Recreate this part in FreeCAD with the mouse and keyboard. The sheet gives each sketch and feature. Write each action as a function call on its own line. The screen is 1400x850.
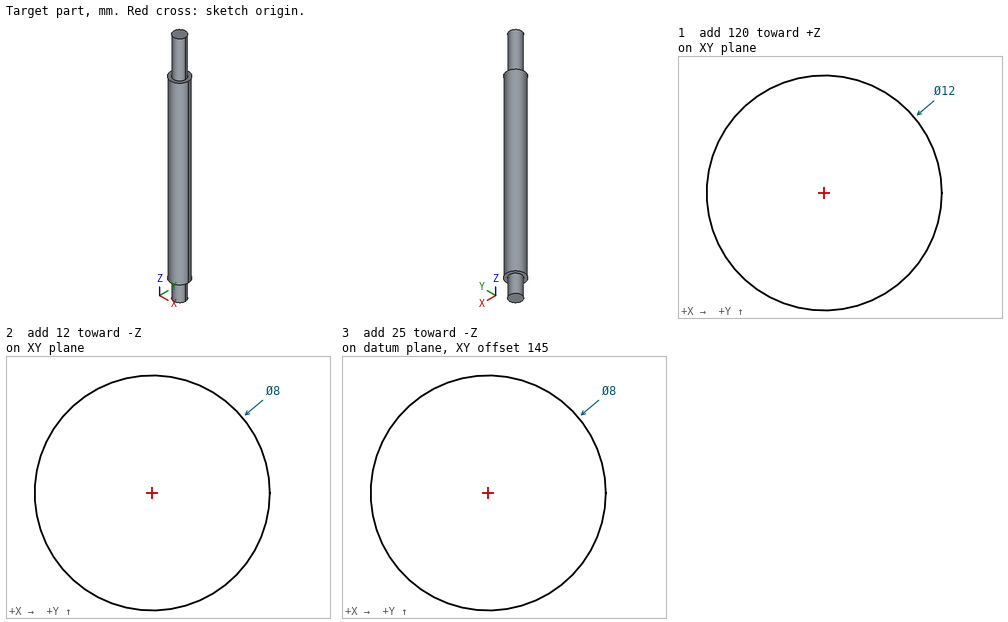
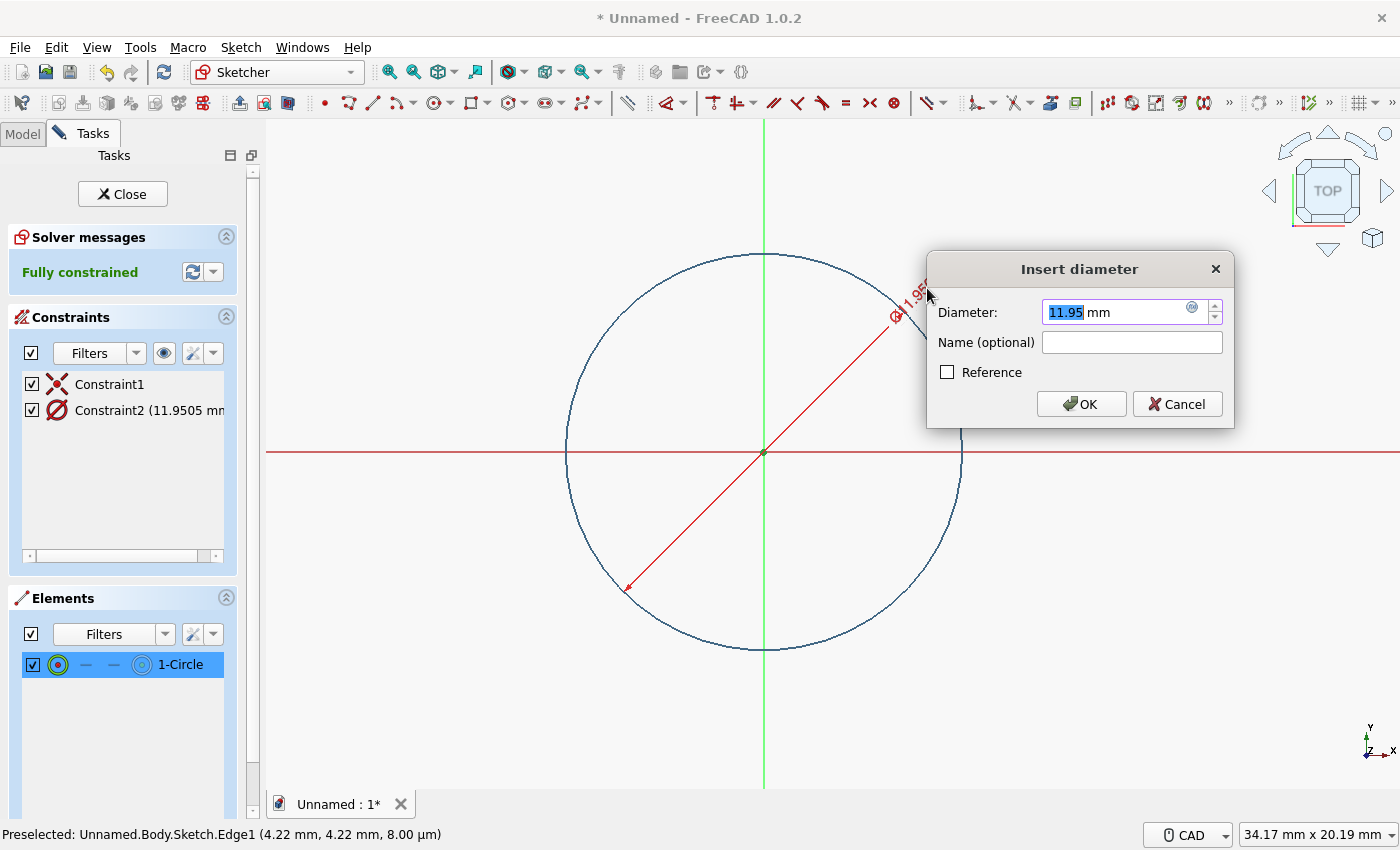
text(12)
key(Return)
key(Escape)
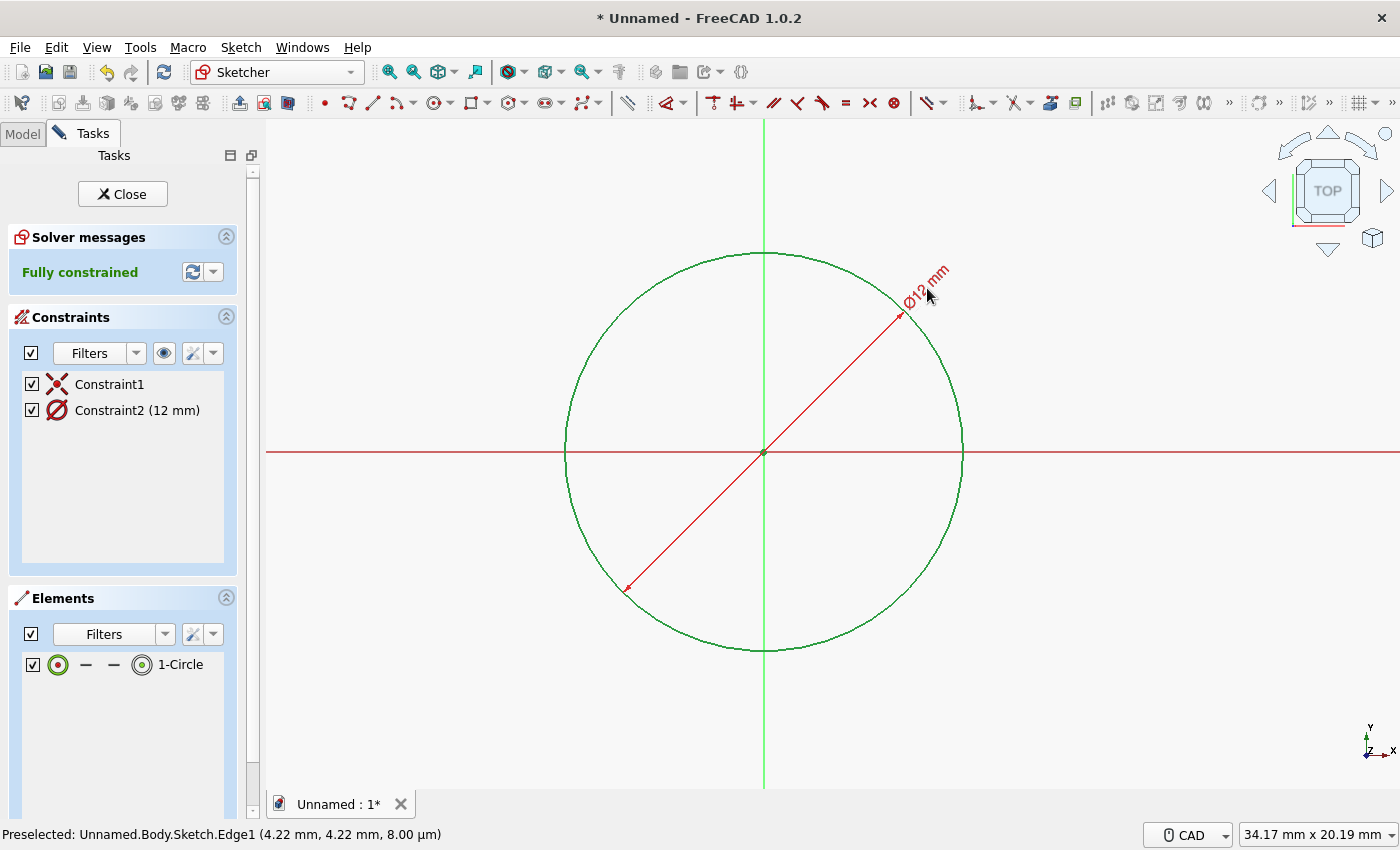
click(123, 194)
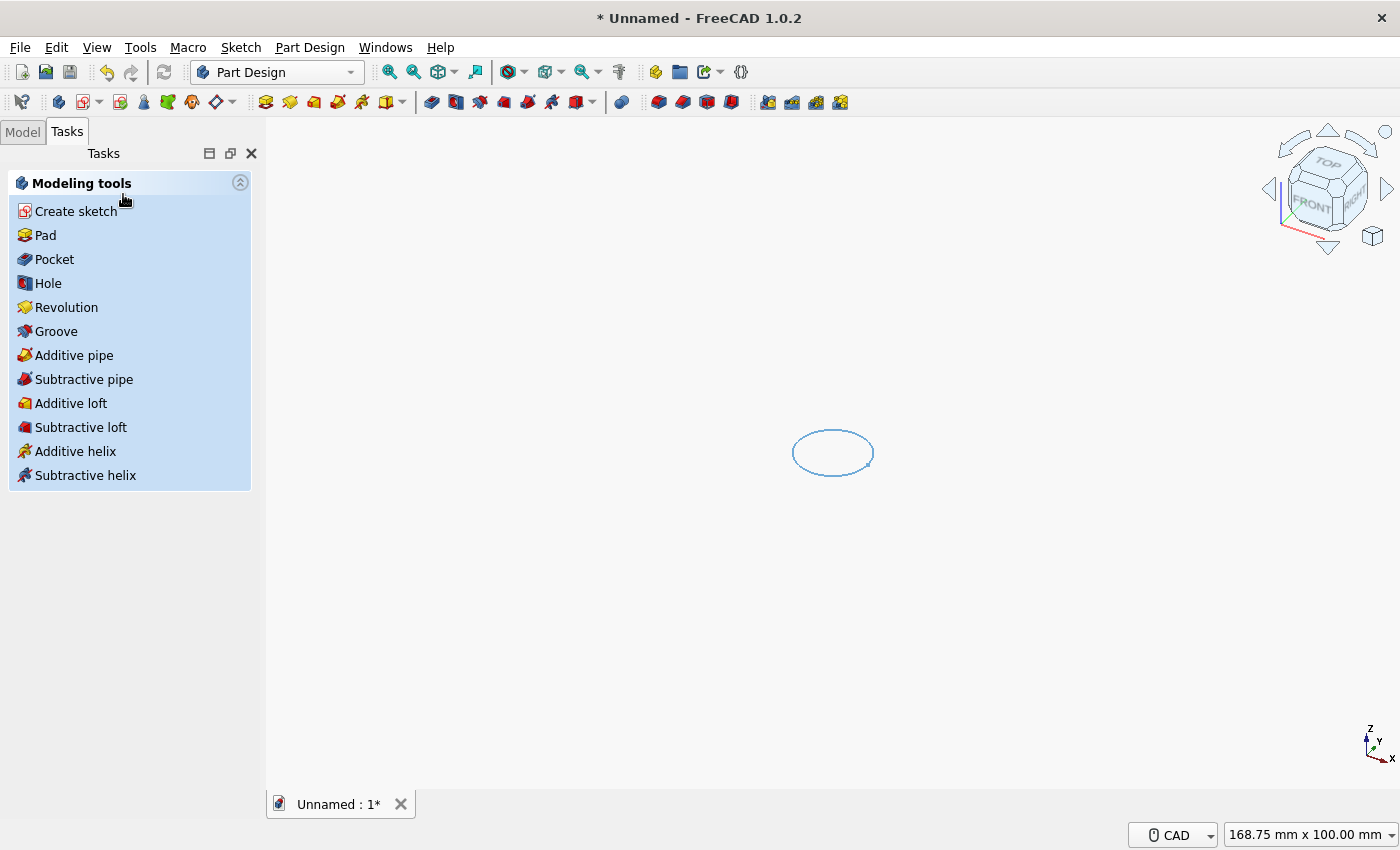
click(266, 102)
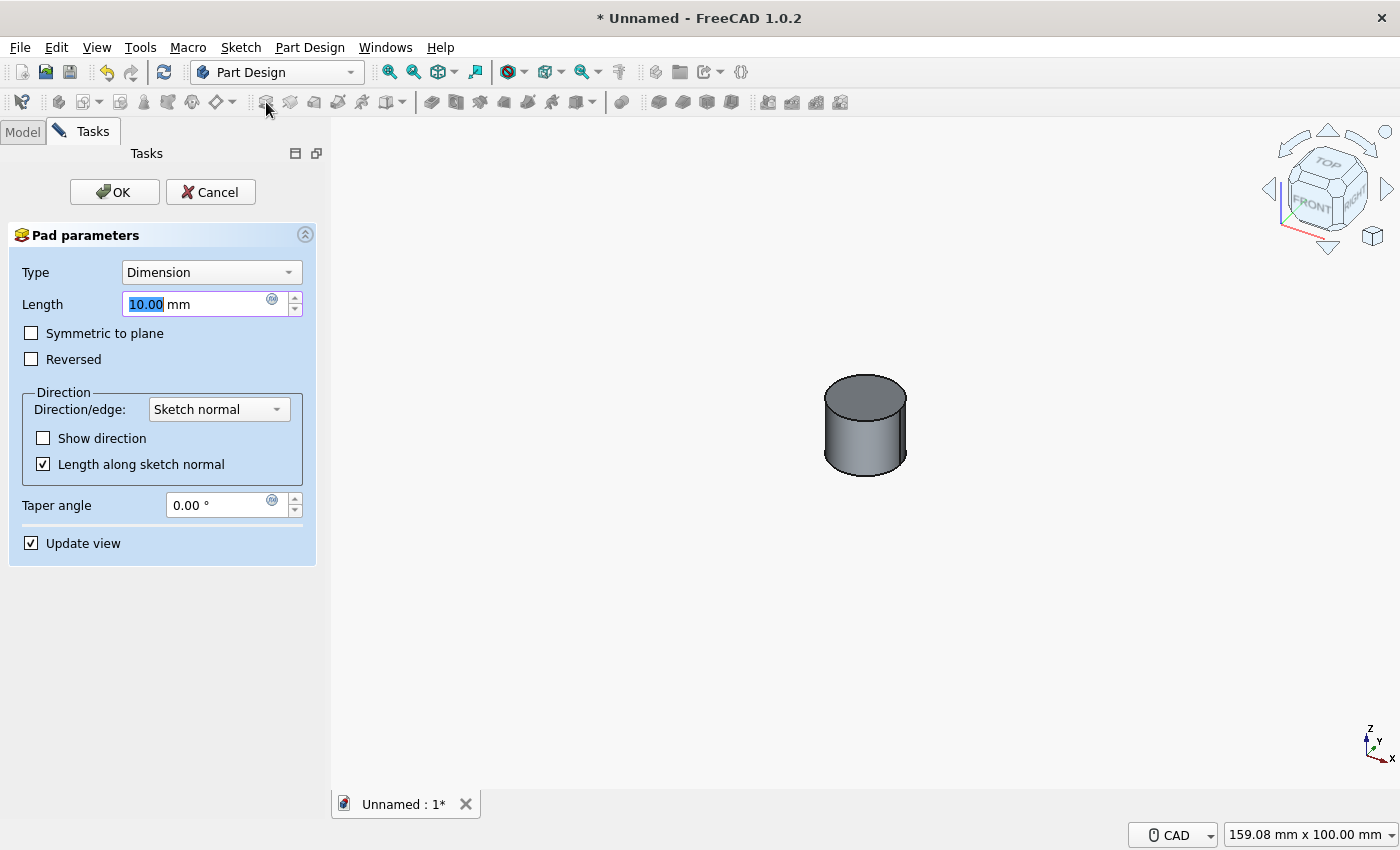
text(120)
key(Tab)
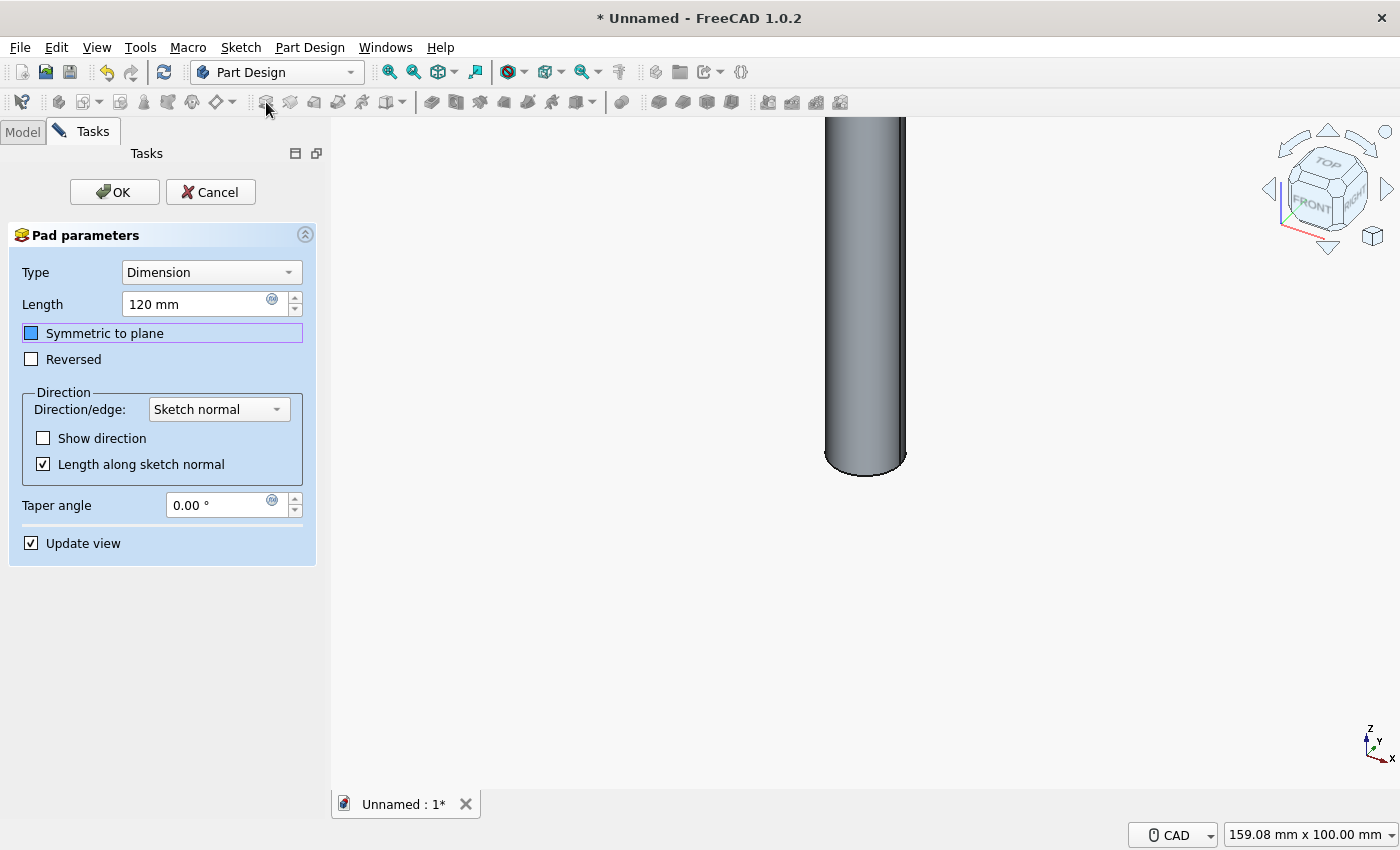
click(115, 192)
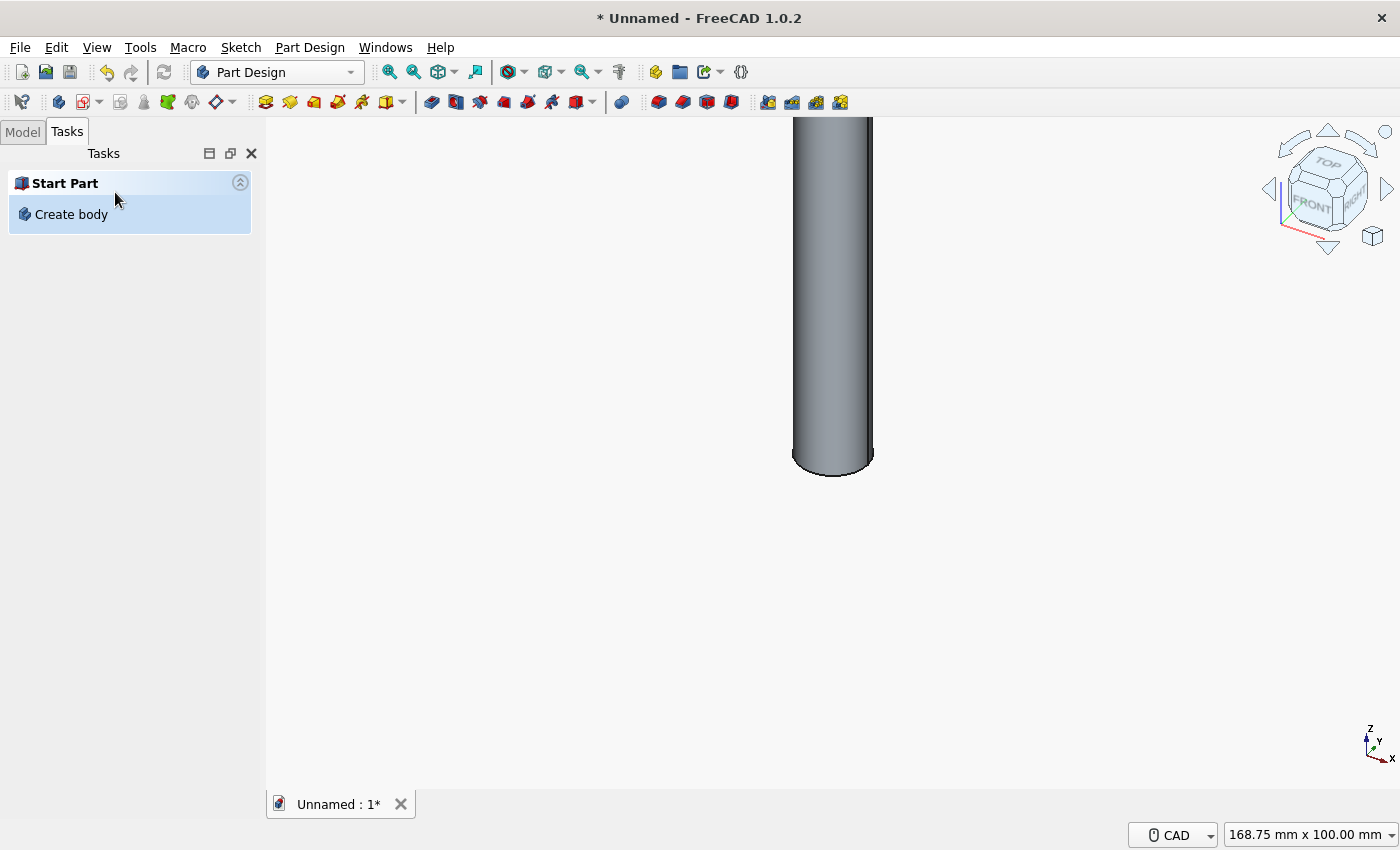
click(390, 72)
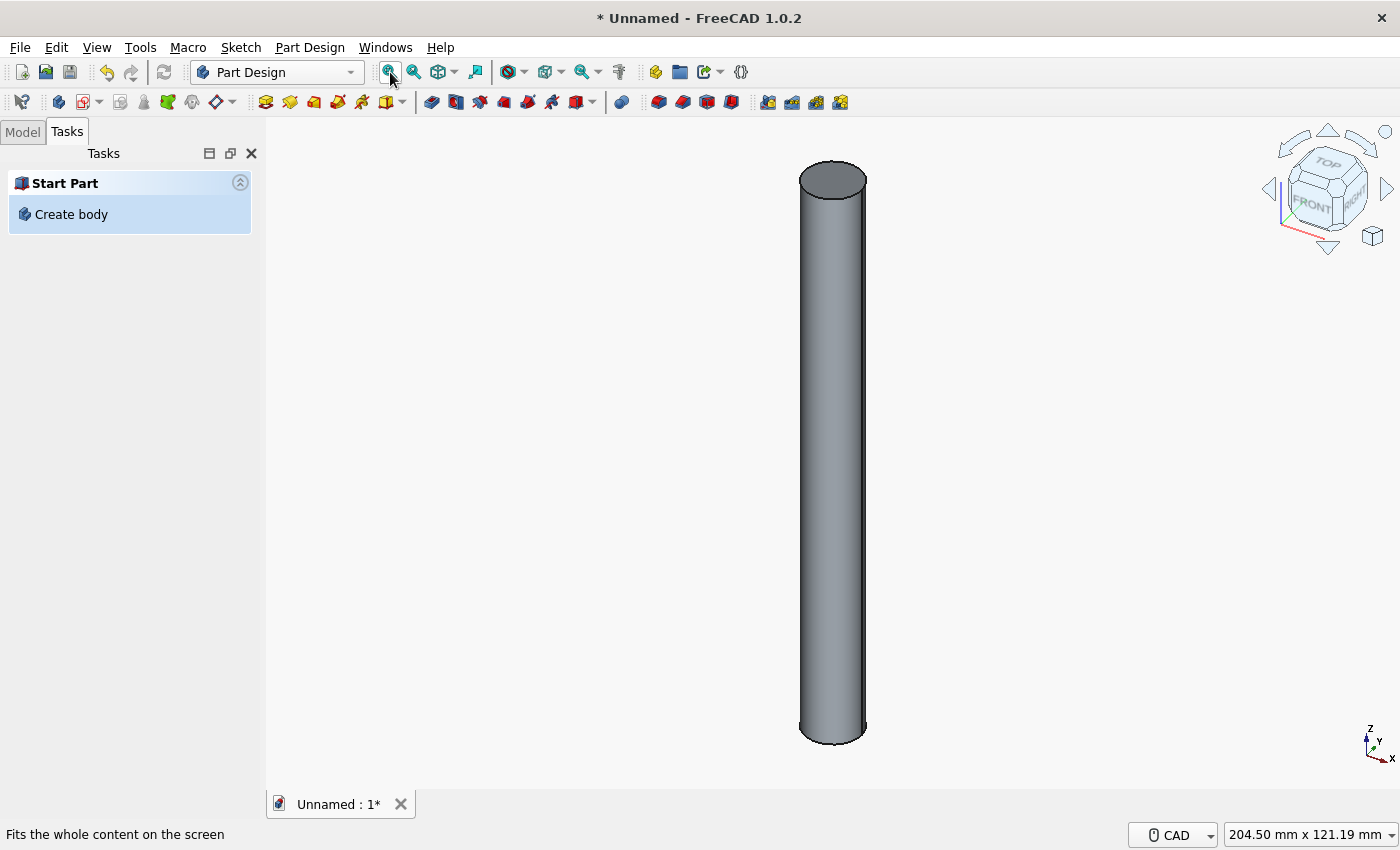
click(84, 102)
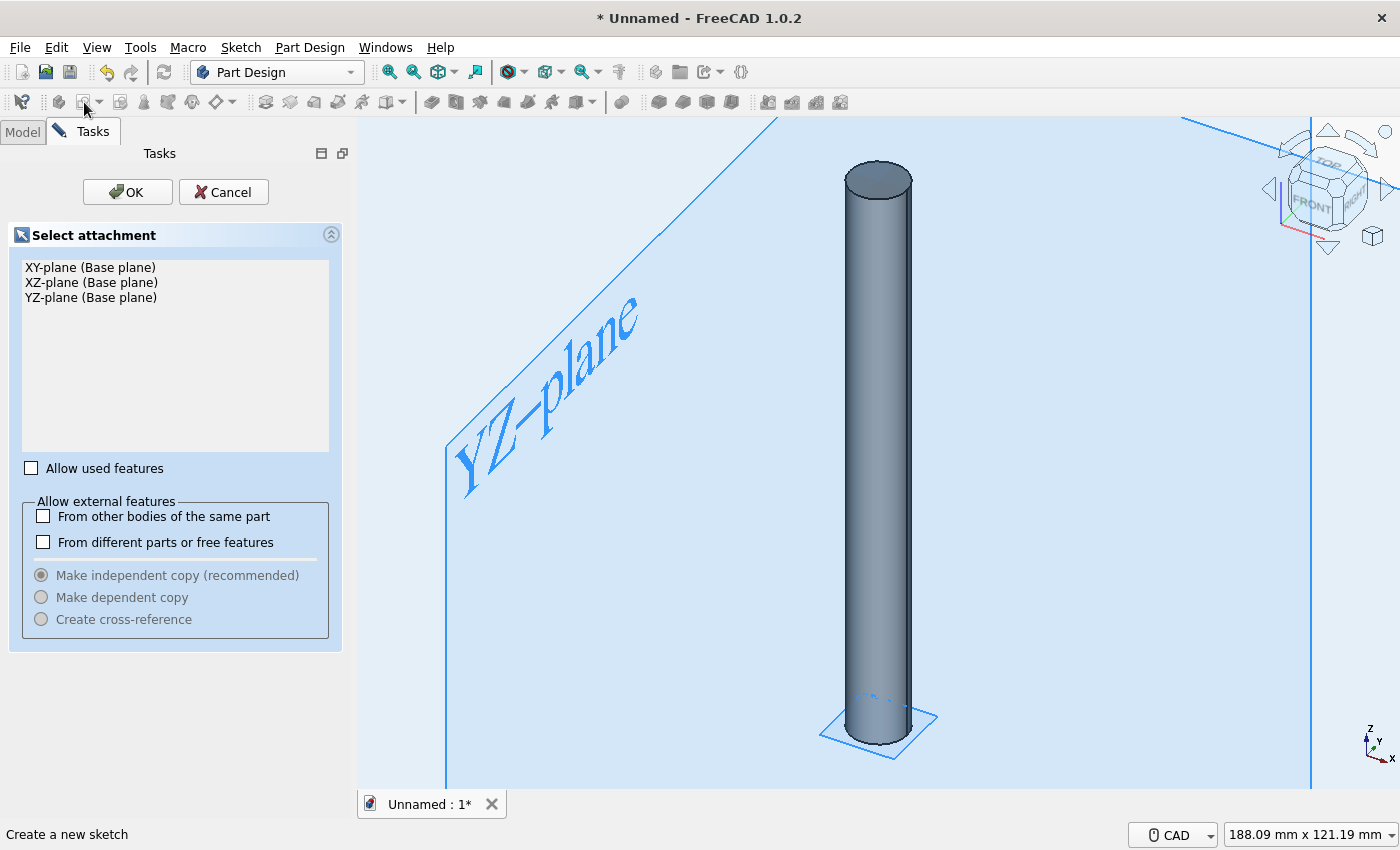
click(82, 268)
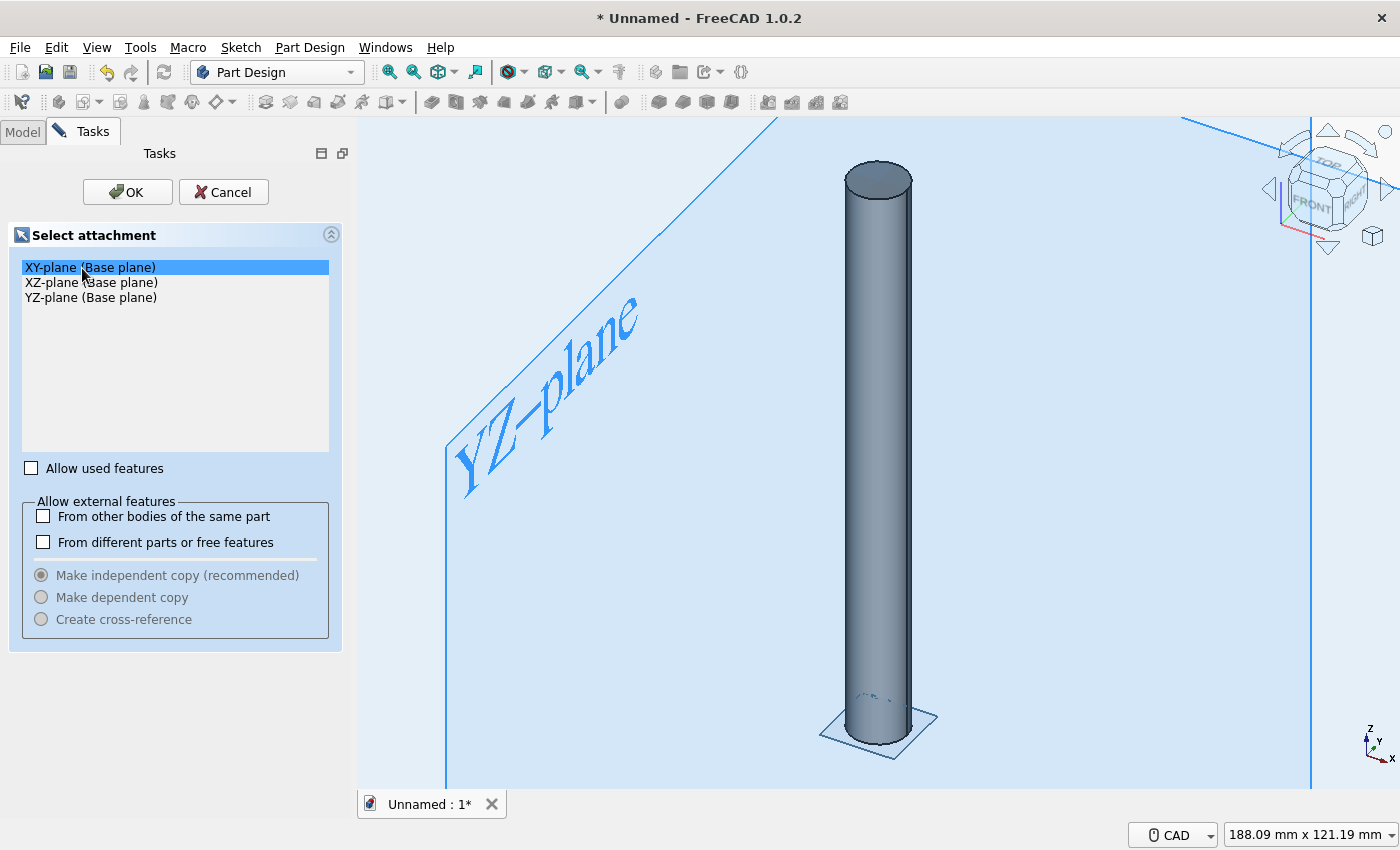
click(128, 192)